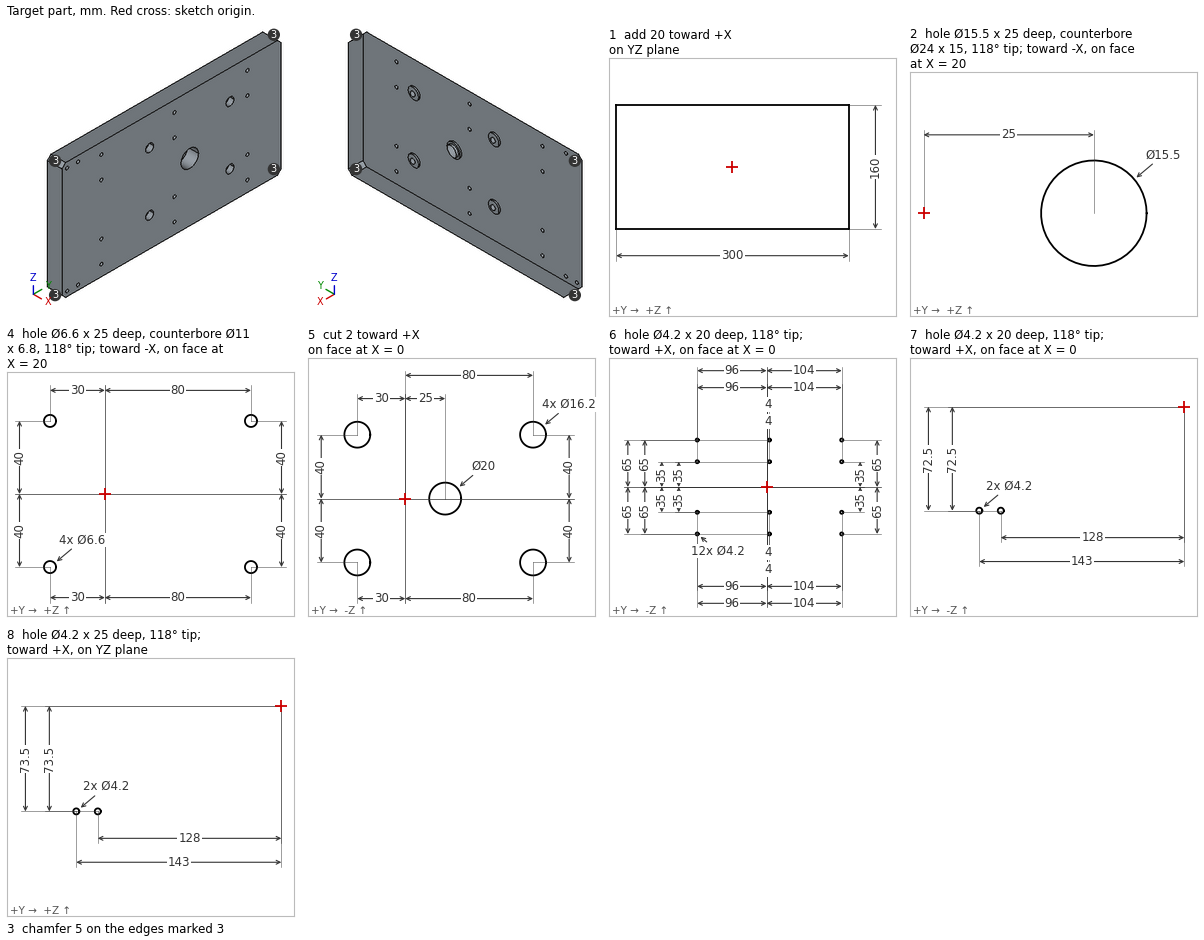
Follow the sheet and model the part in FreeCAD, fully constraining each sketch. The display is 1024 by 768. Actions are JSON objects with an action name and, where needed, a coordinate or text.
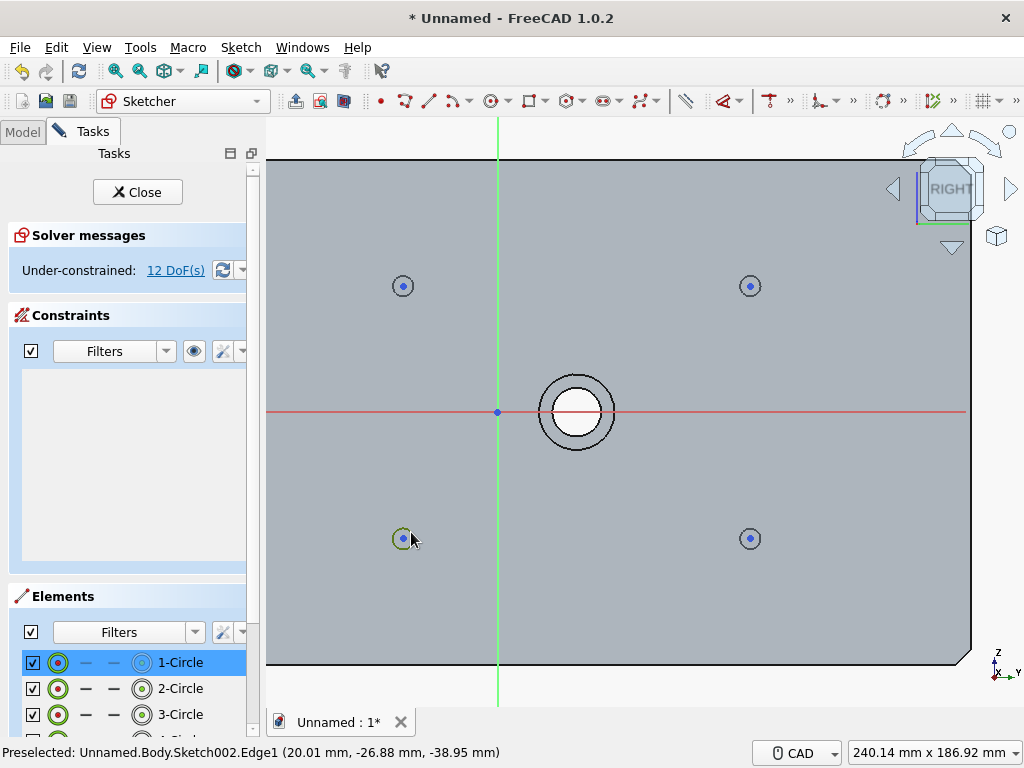
{"action": "scroll", "coordinate": [758, 532], "scroll_direction": "up", "scroll_amount": 2}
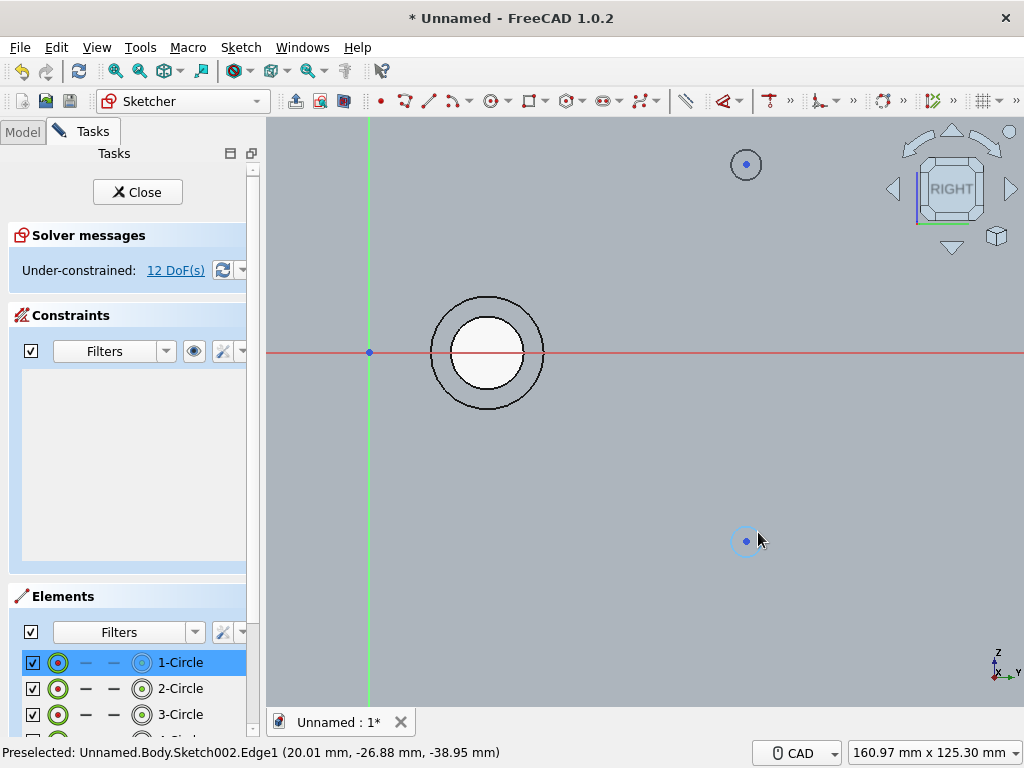
{"action": "left_click", "coordinate": [757, 531]}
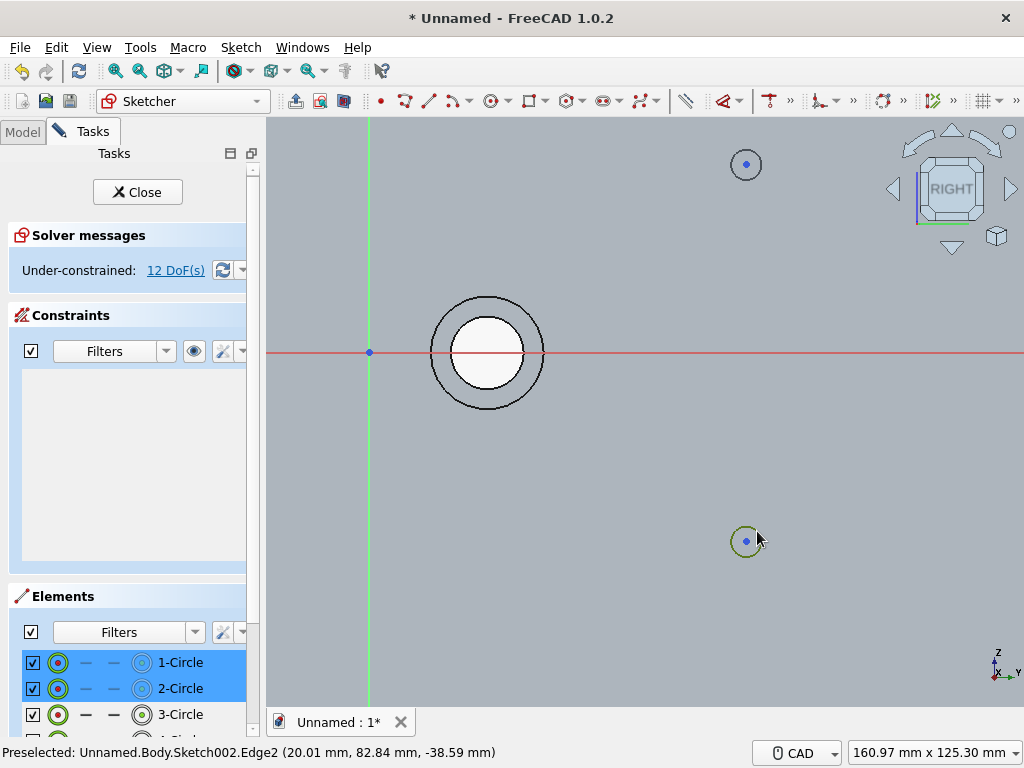
{"action": "scroll", "coordinate": [758, 532], "scroll_direction": "down", "scroll_amount": 2}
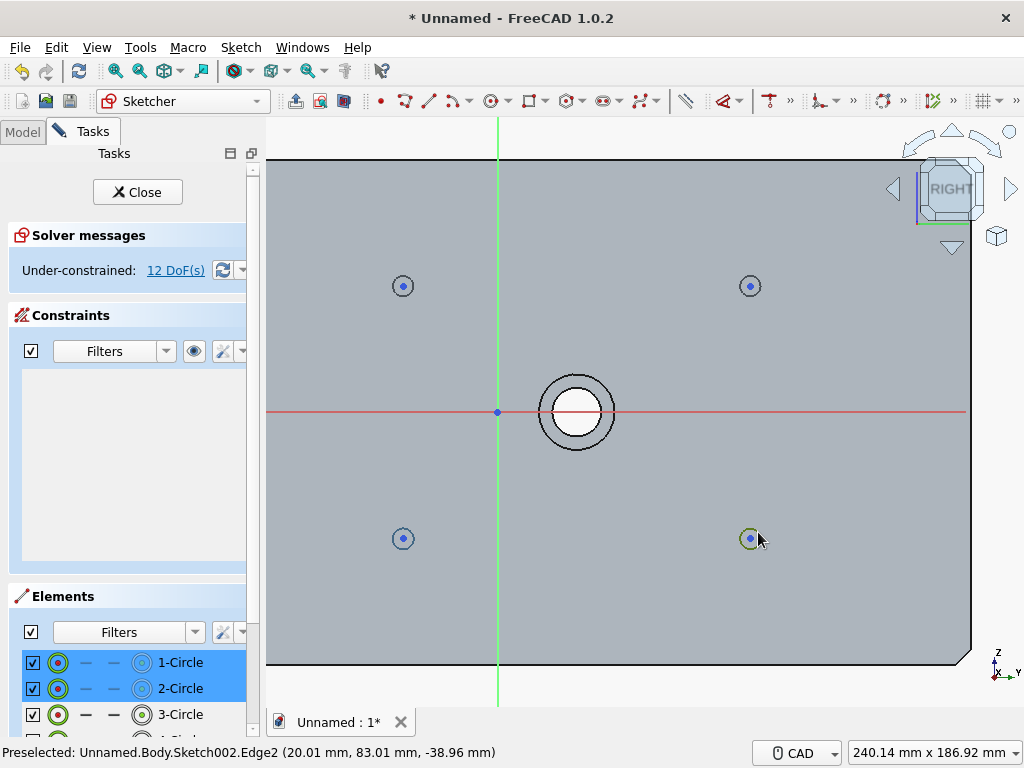
{"action": "scroll", "coordinate": [410, 279], "scroll_direction": "up", "scroll_amount": 2}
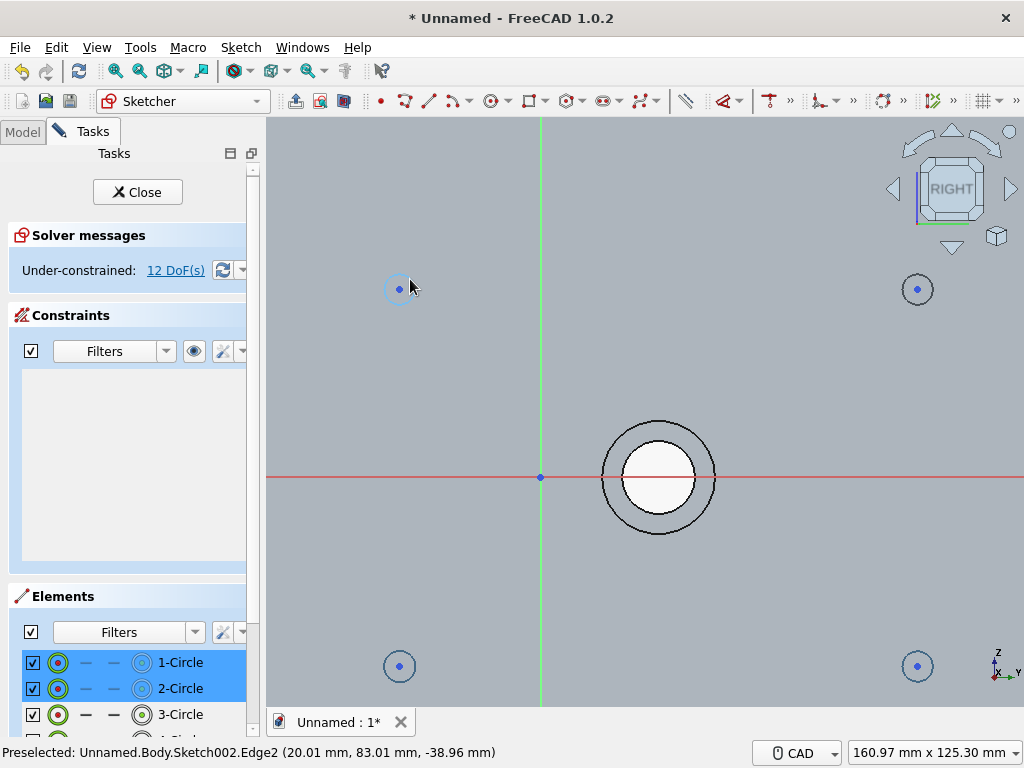
{"action": "left_click", "coordinate": [410, 279]}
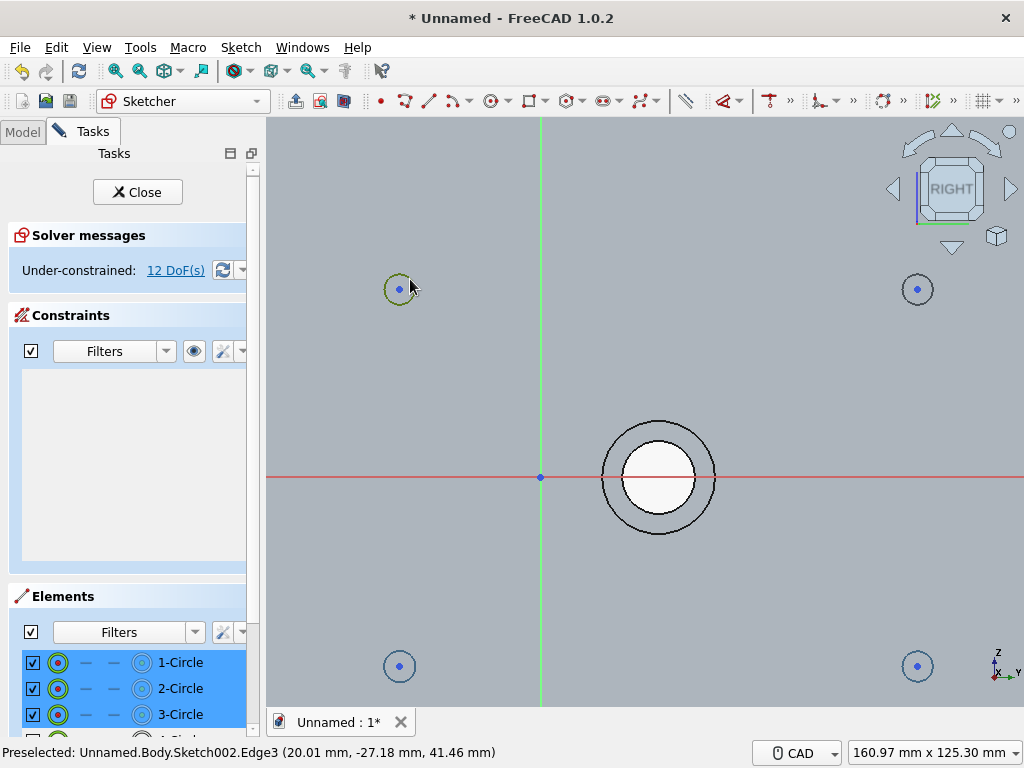
{"action": "scroll", "coordinate": [410, 279], "scroll_direction": "down", "scroll_amount": 2}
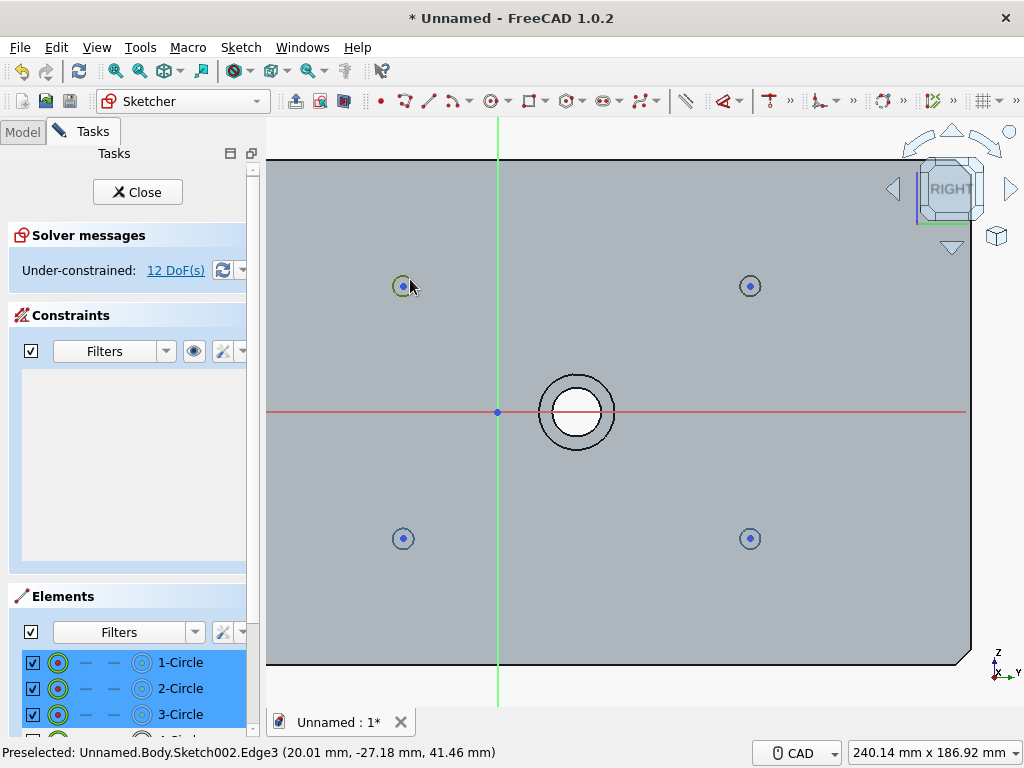
{"action": "scroll", "coordinate": [758, 279], "scroll_direction": "up", "scroll_amount": 2}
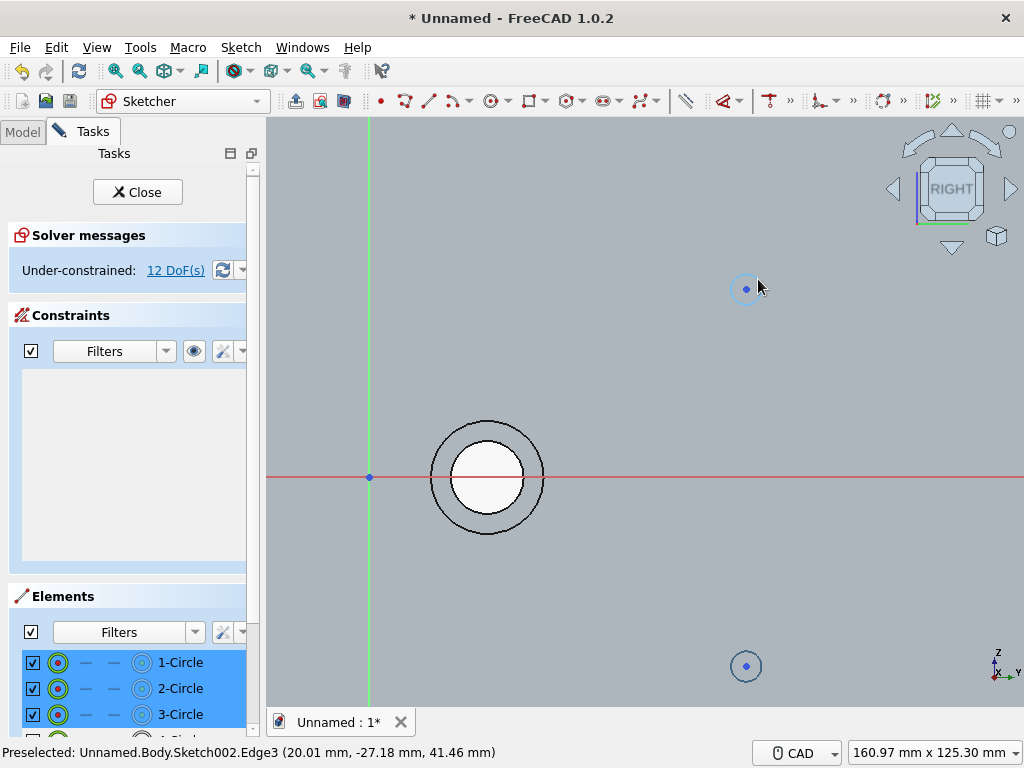
{"action": "left_click", "coordinate": [757, 279]}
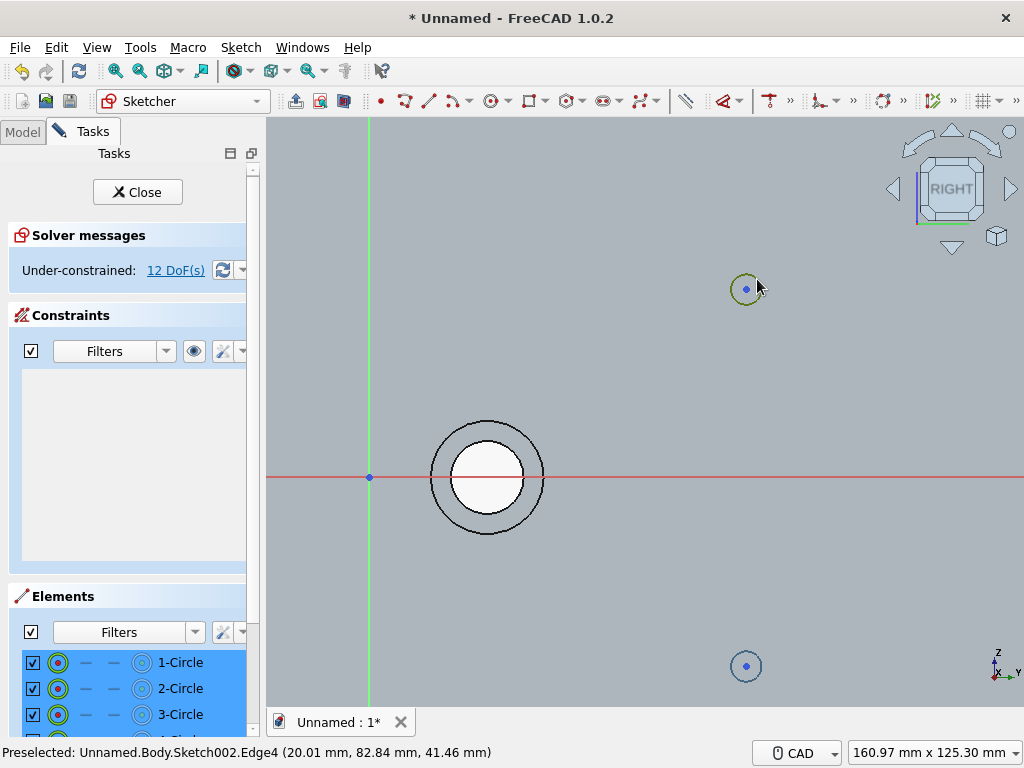
{"action": "key", "text": "e"}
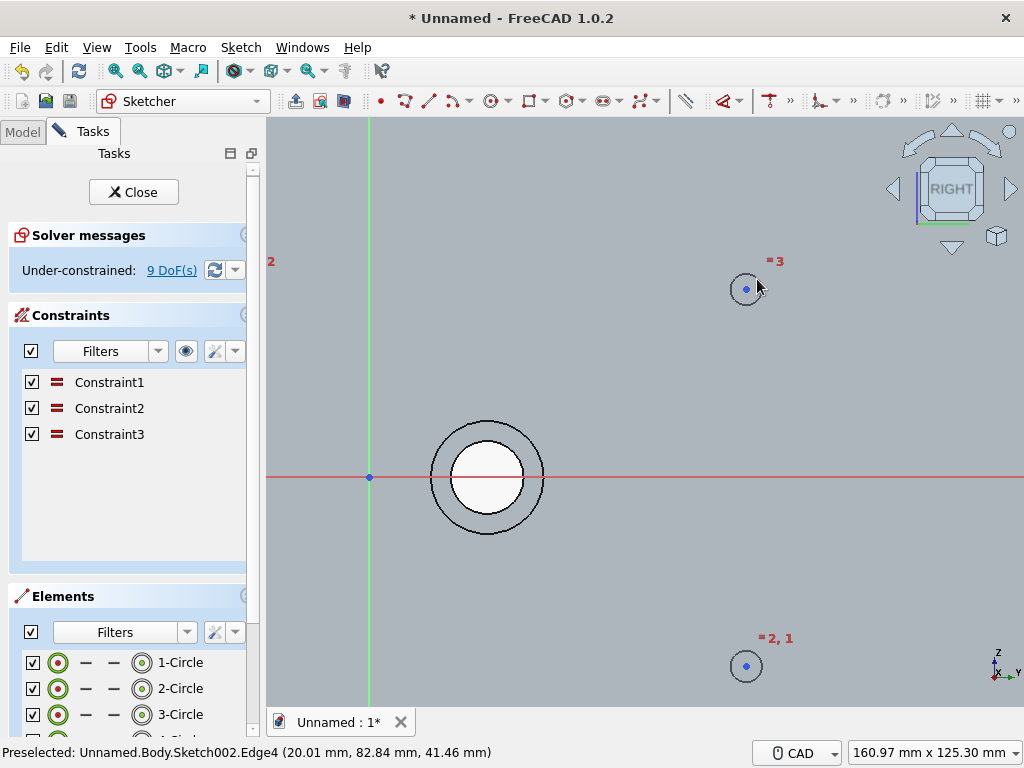
{"action": "key", "text": "d"}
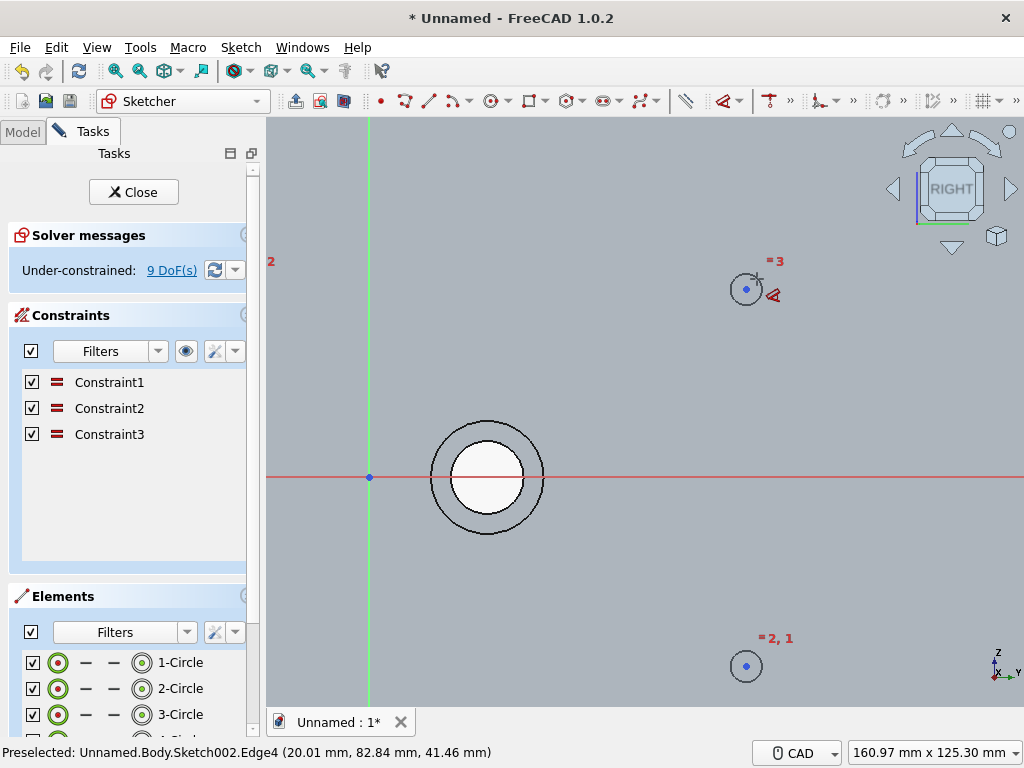
{"action": "scroll", "coordinate": [758, 279], "scroll_direction": "down", "scroll_amount": 2}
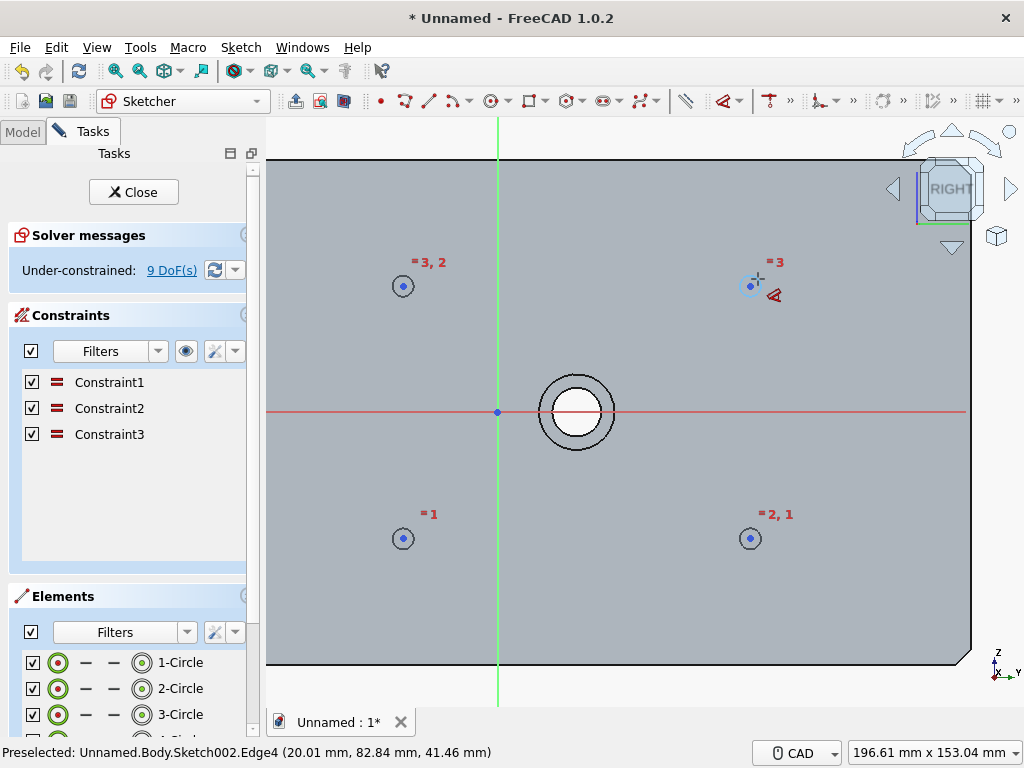
{"action": "scroll", "coordinate": [411, 532], "scroll_direction": "up", "scroll_amount": 4}